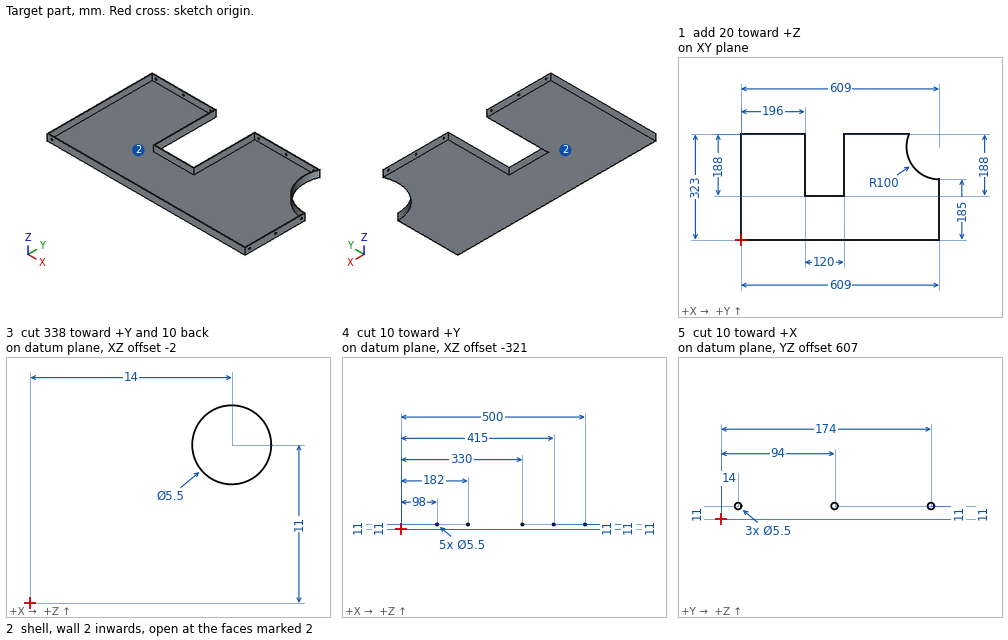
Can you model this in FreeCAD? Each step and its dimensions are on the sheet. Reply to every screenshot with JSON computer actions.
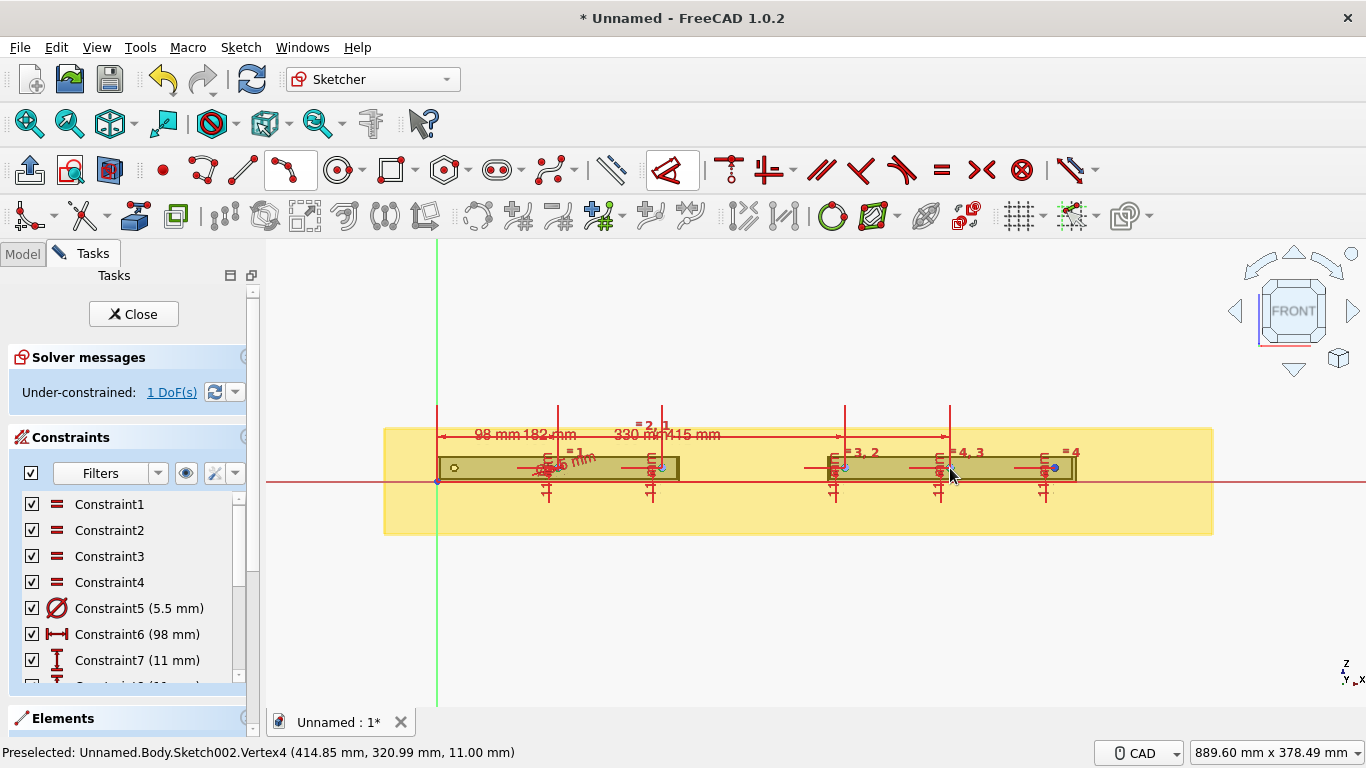
{"action": "left_click", "coordinate": [1055, 468]}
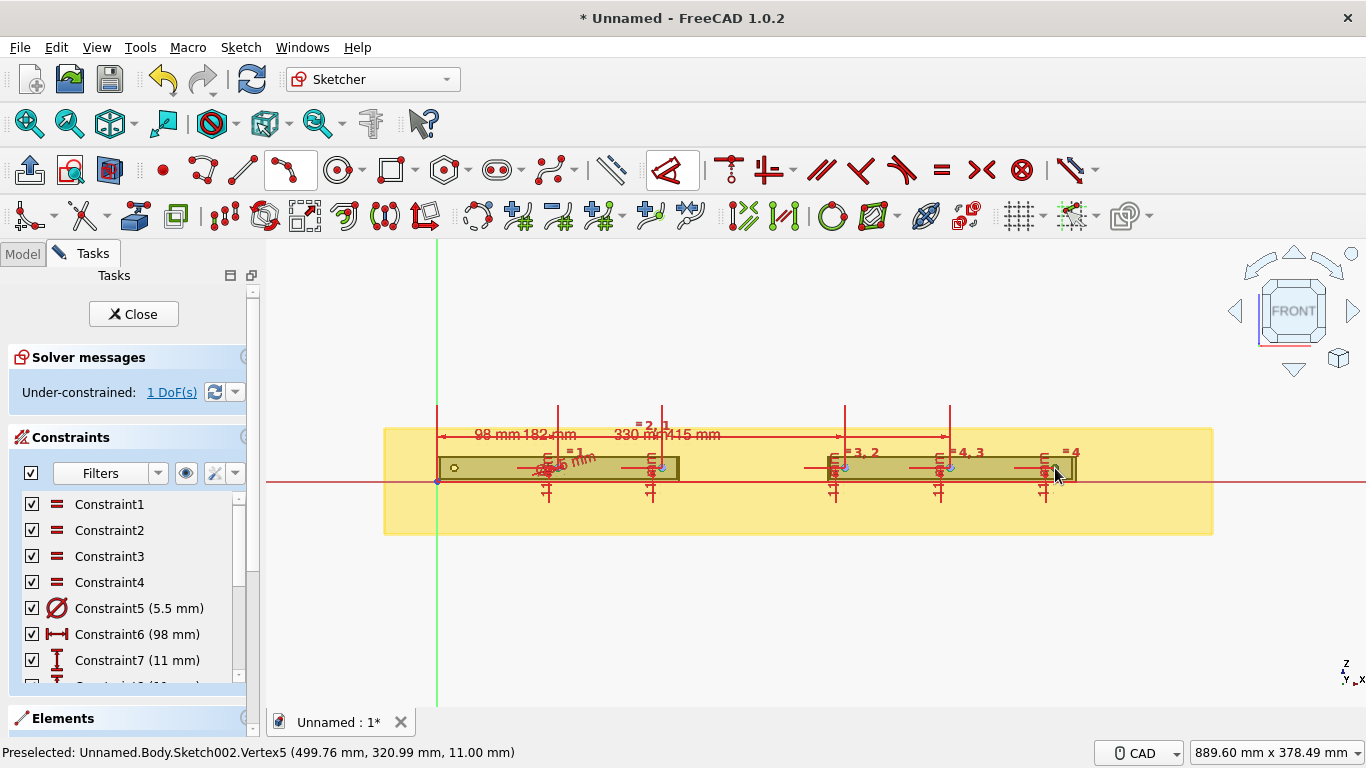
{"action": "key", "text": "l"}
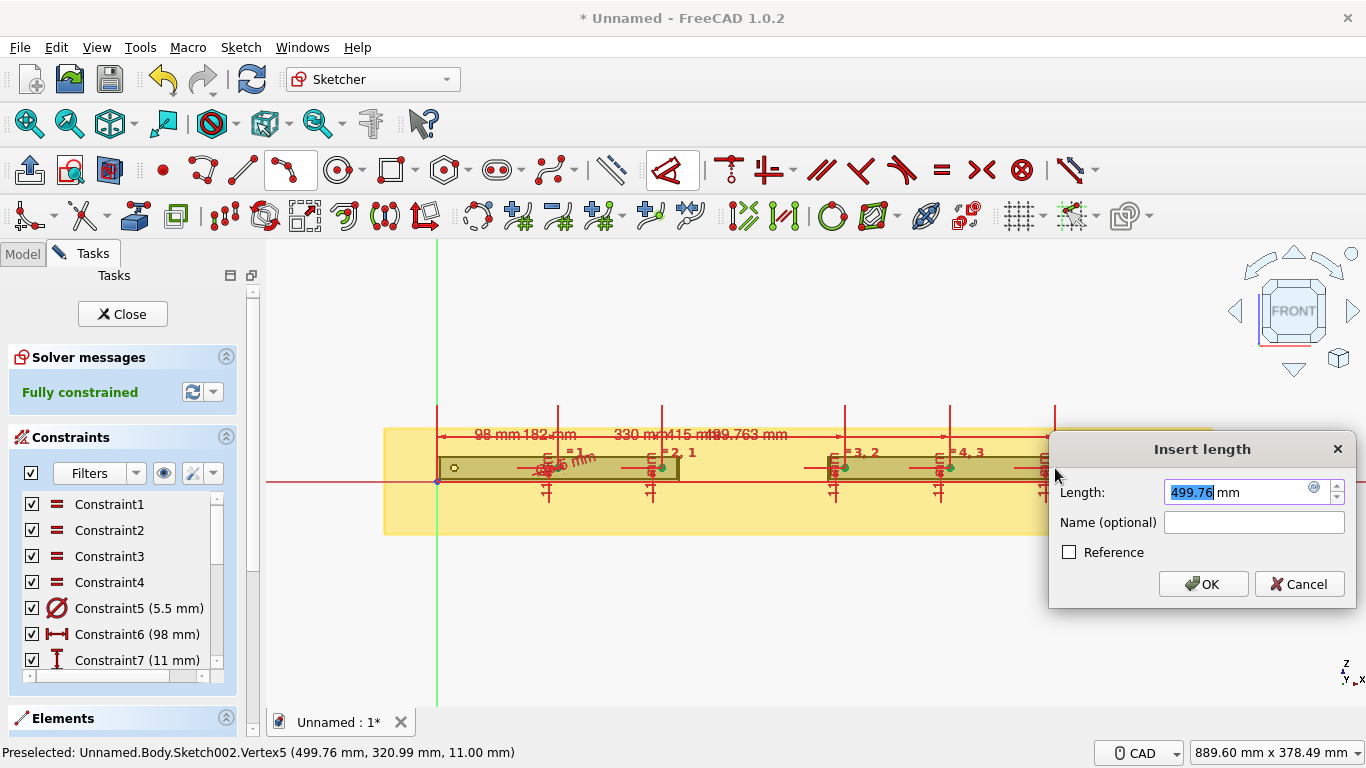
{"action": "type", "text": "500"}
{"action": "key", "text": "Return"}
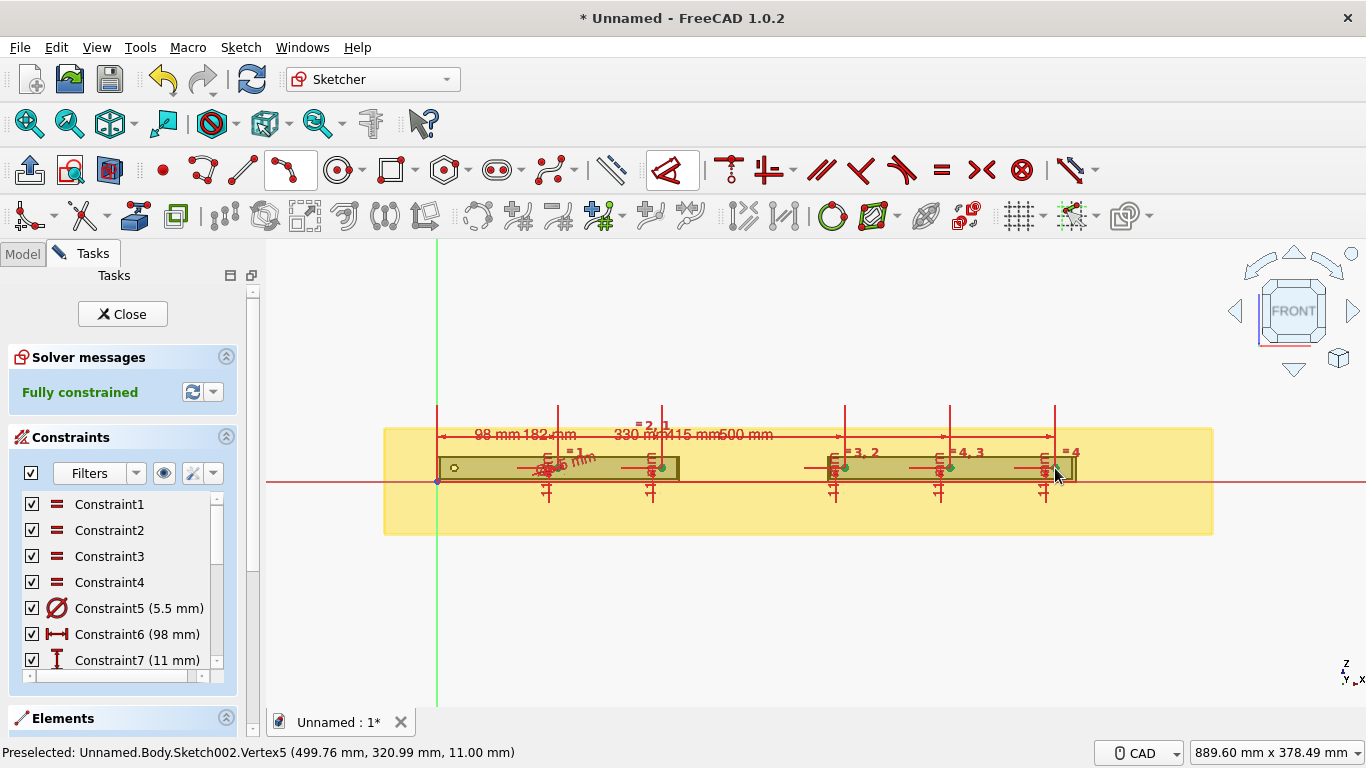
{"action": "left_click", "coordinate": [123, 314]}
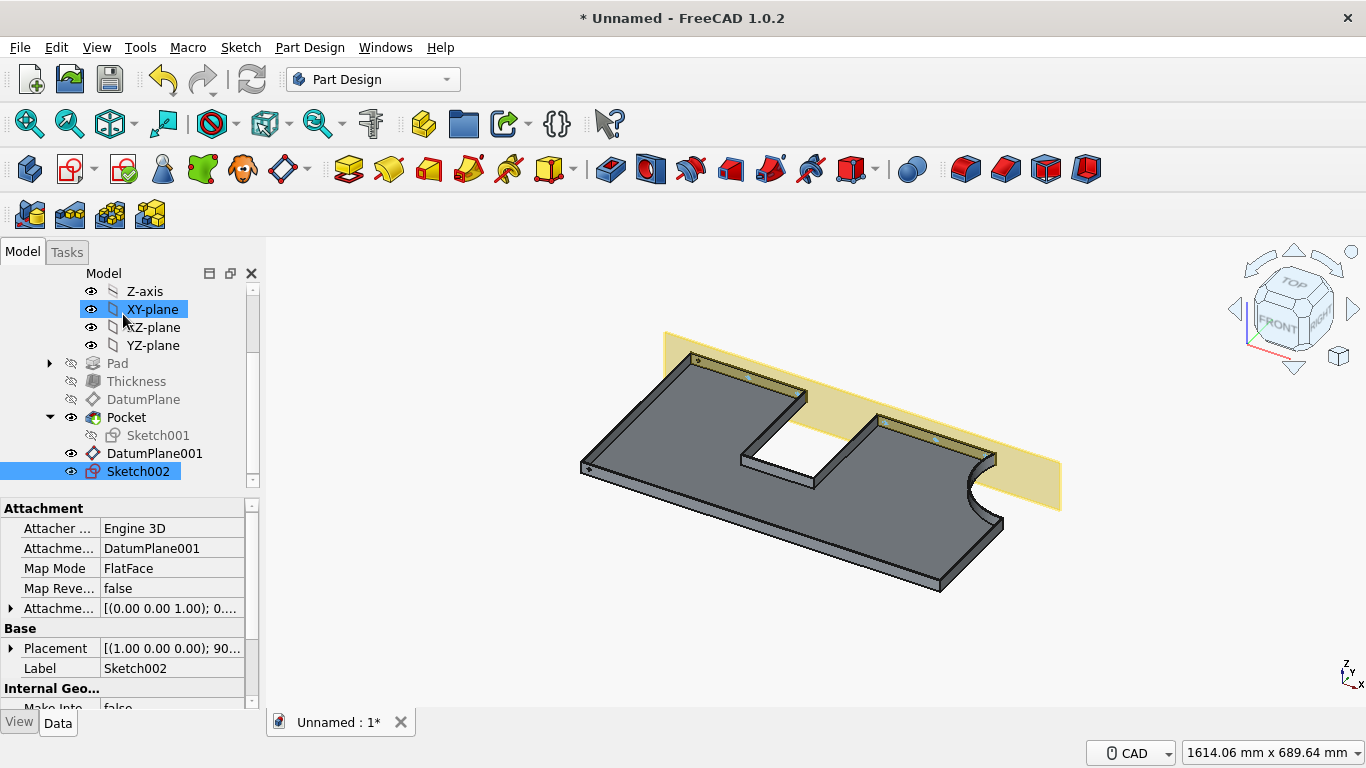
{"action": "left_click", "coordinate": [612, 170]}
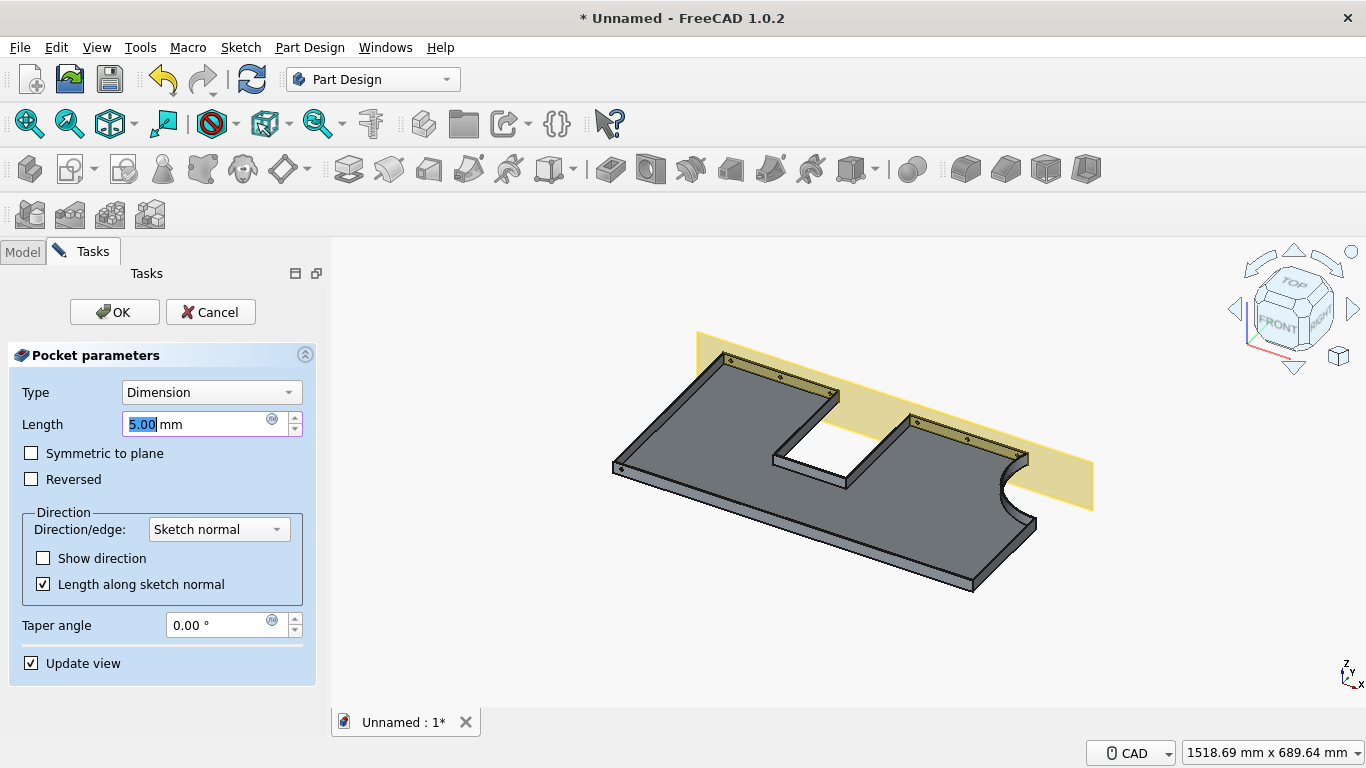
{"action": "type", "text": "10"}
{"action": "key", "text": "Tab"}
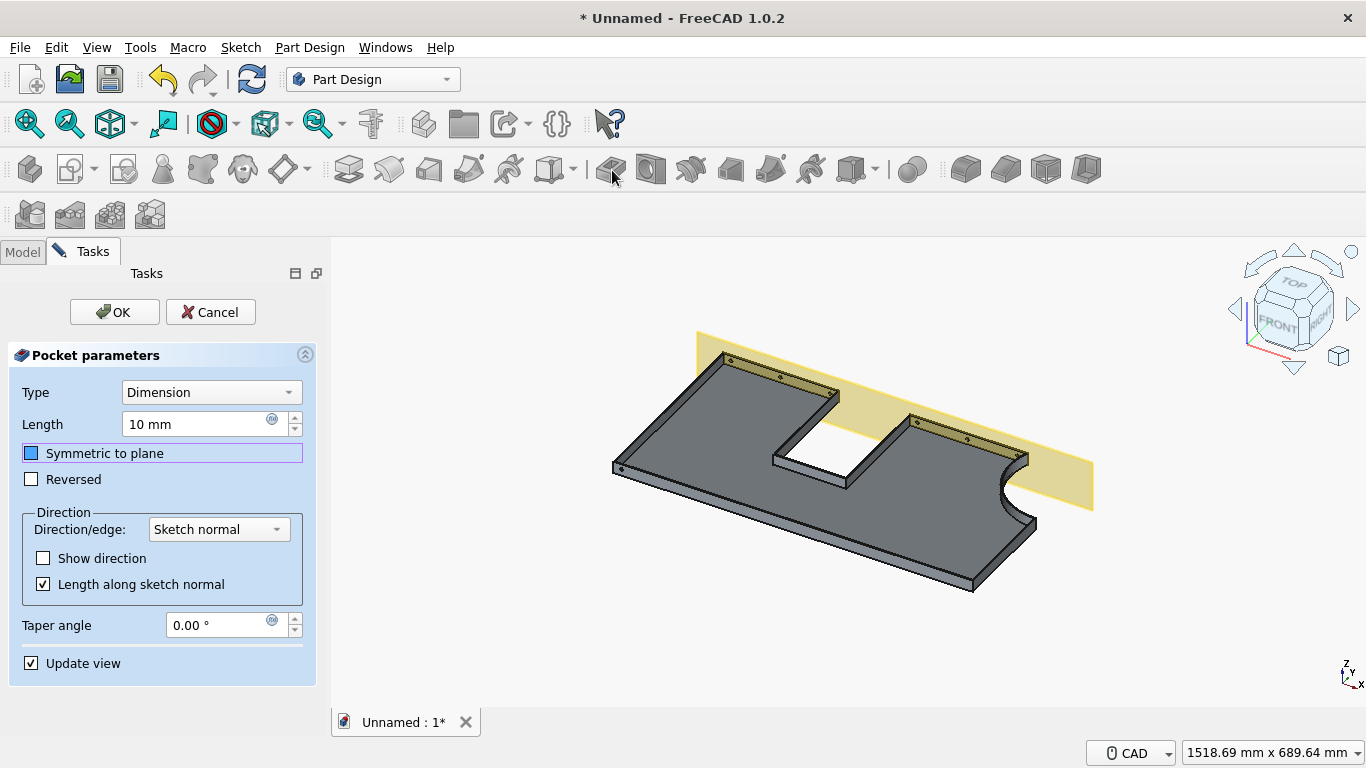
{"action": "left_click", "coordinate": [115, 312]}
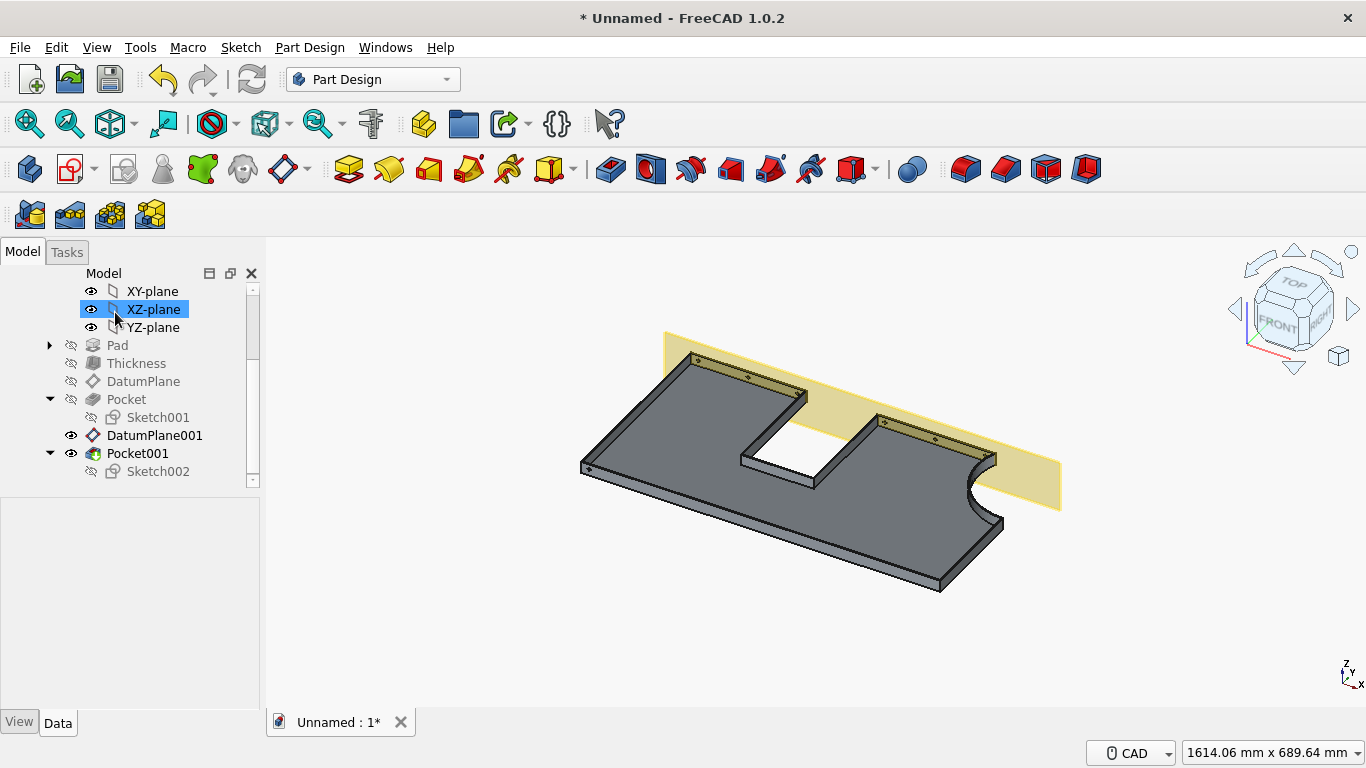
{"action": "left_click", "coordinate": [116, 435]}
{"action": "key", "text": "space"}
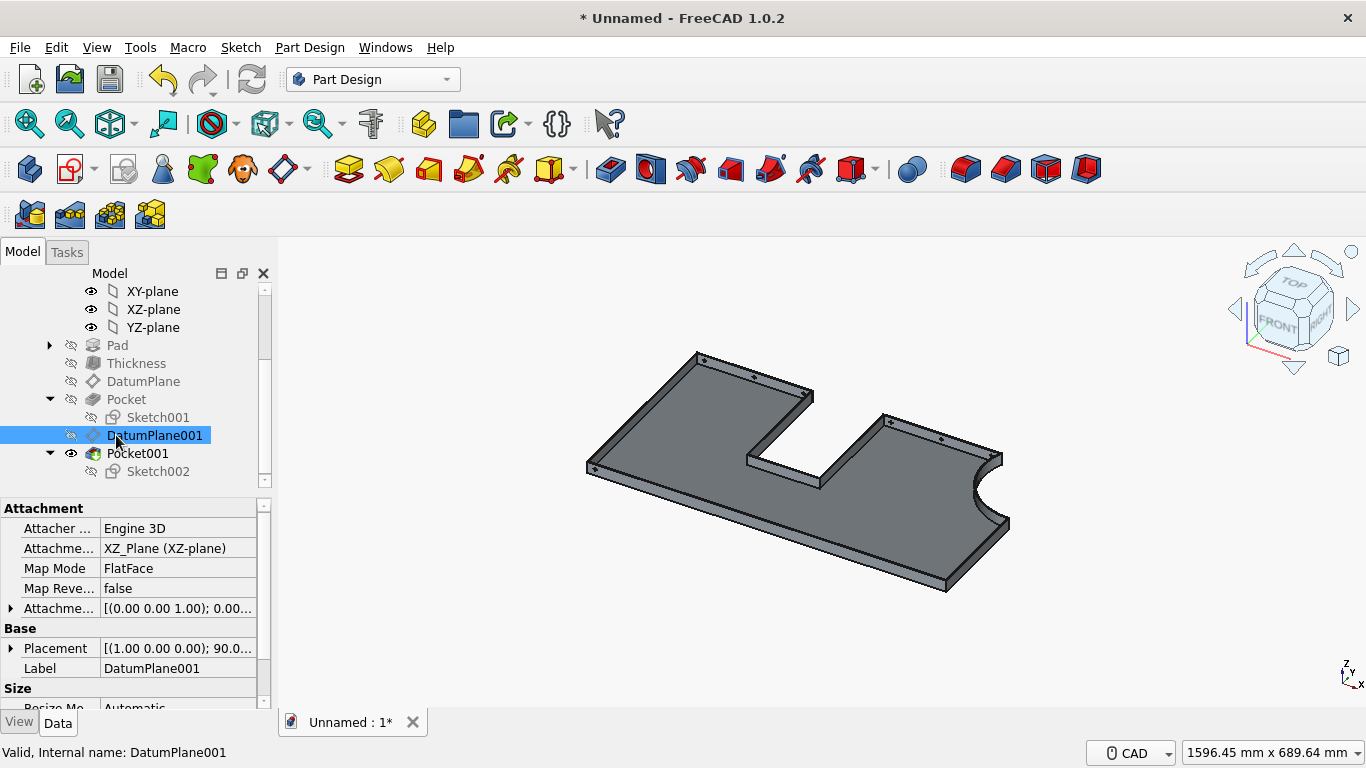
{"action": "scroll", "coordinate": [160, 377], "scroll_direction": "down", "scroll_amount": 3}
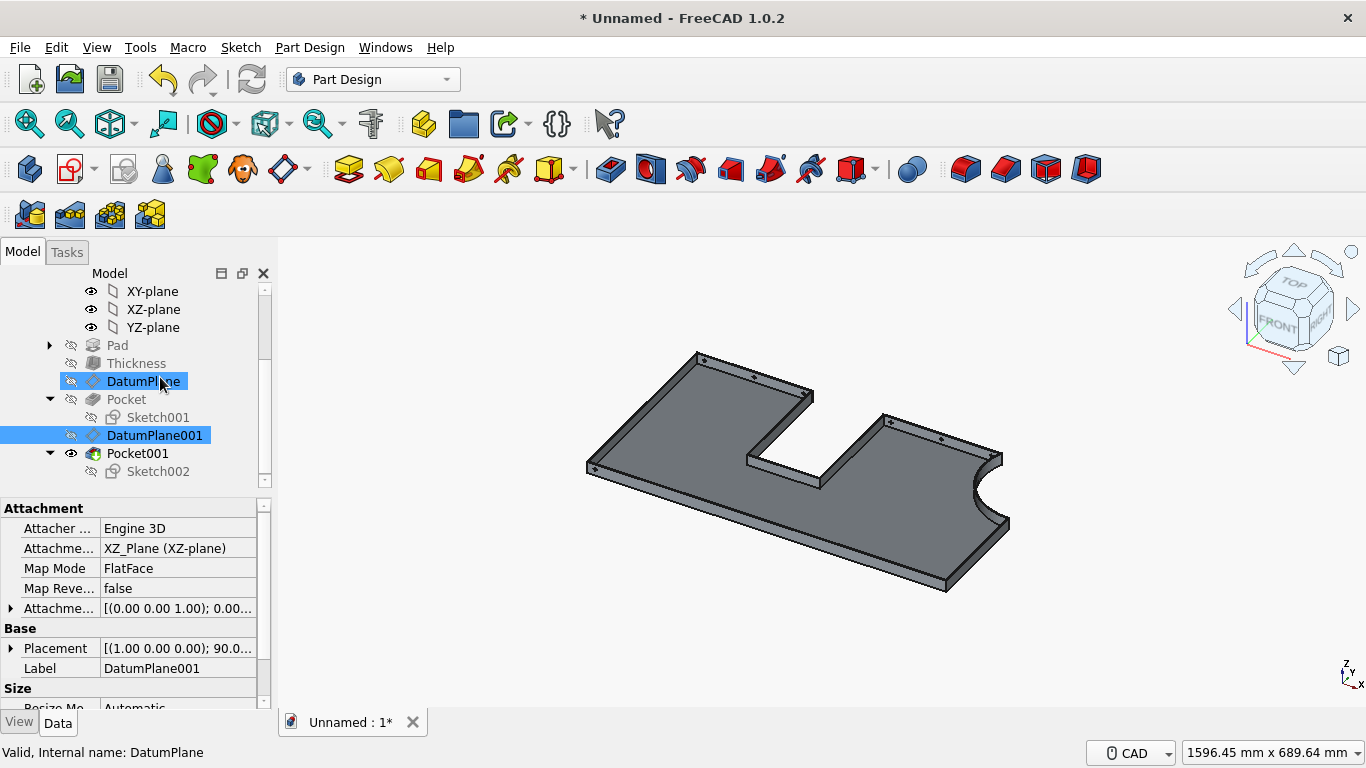
{"action": "scroll", "coordinate": [160, 377], "scroll_direction": "up", "scroll_amount": 15}